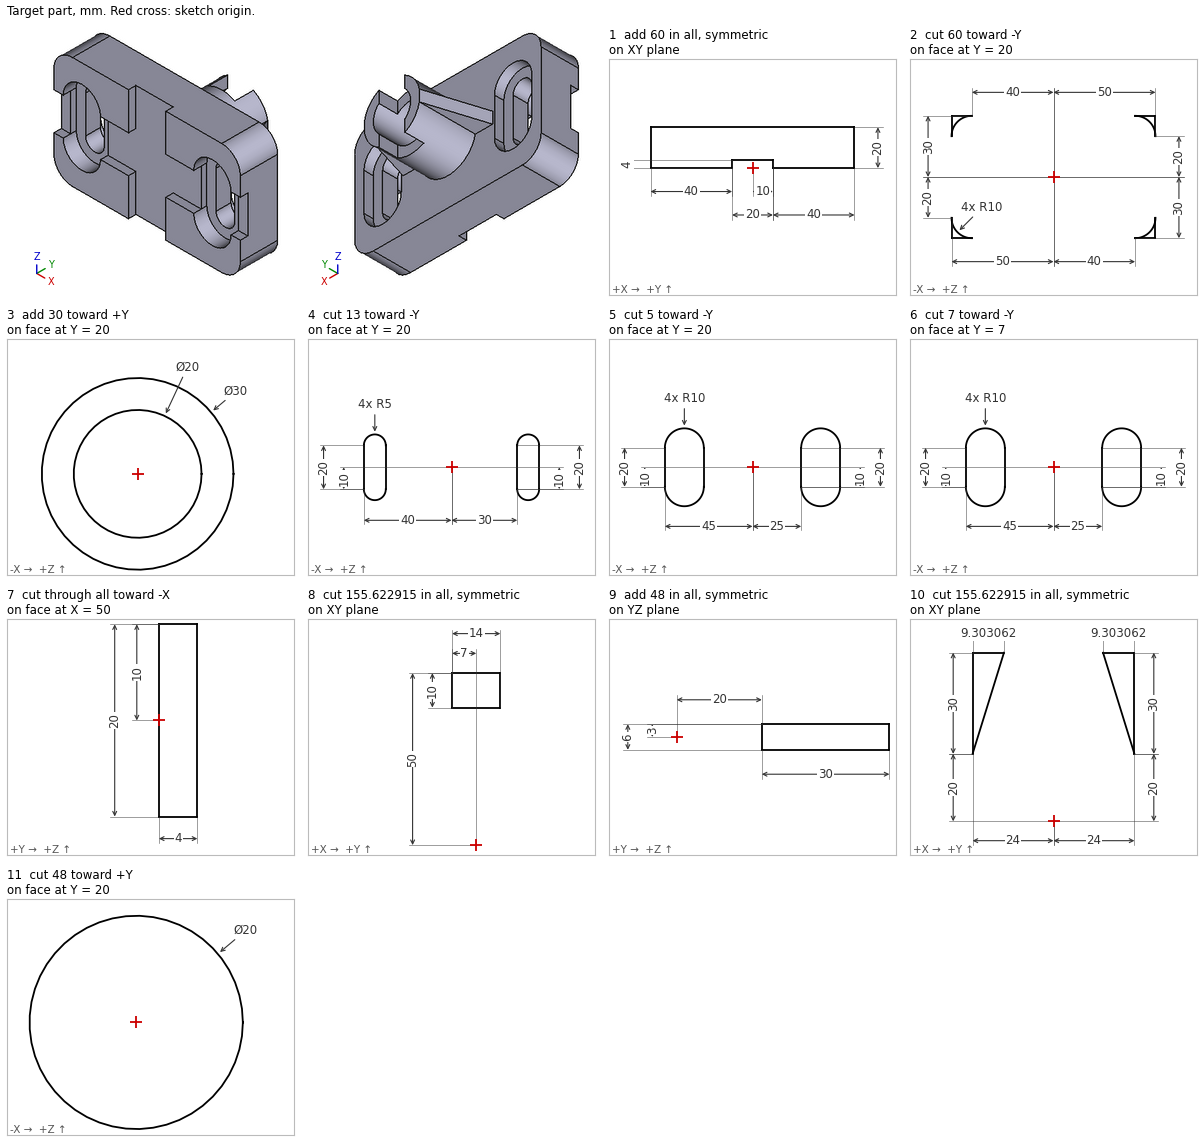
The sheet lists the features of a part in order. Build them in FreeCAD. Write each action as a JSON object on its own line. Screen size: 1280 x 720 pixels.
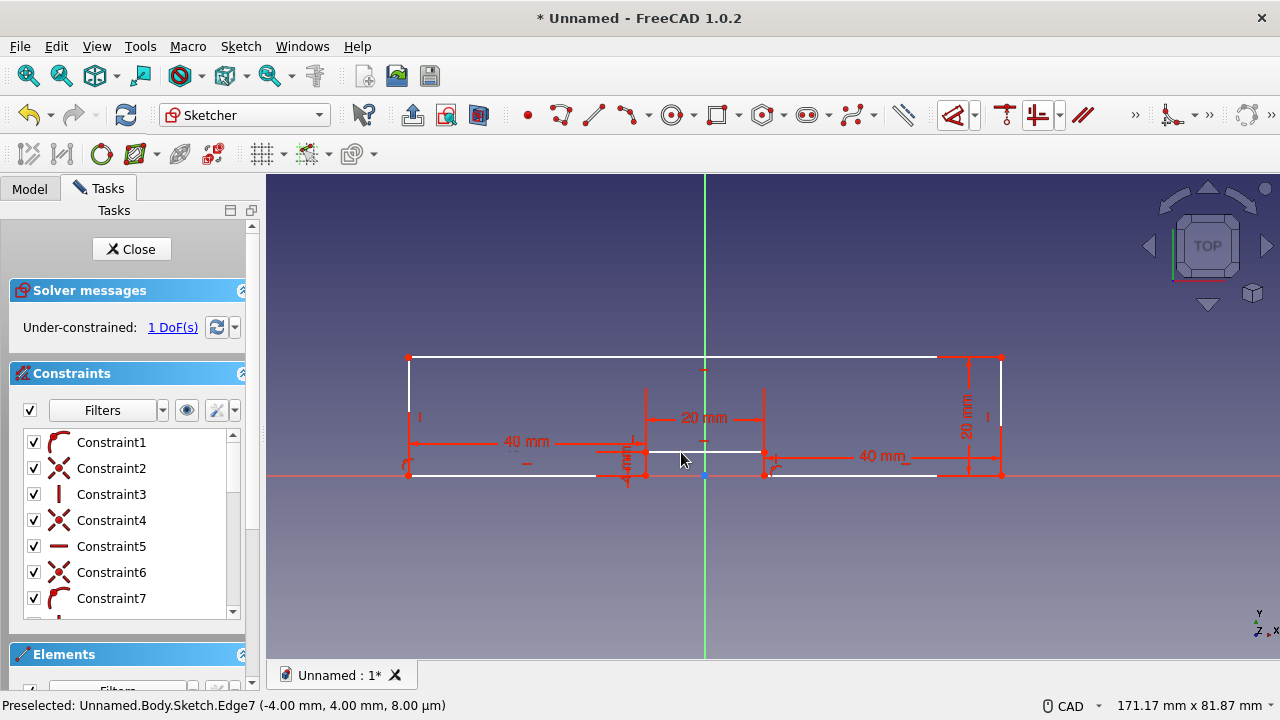
{"action": "left_click", "coordinate": [764, 476]}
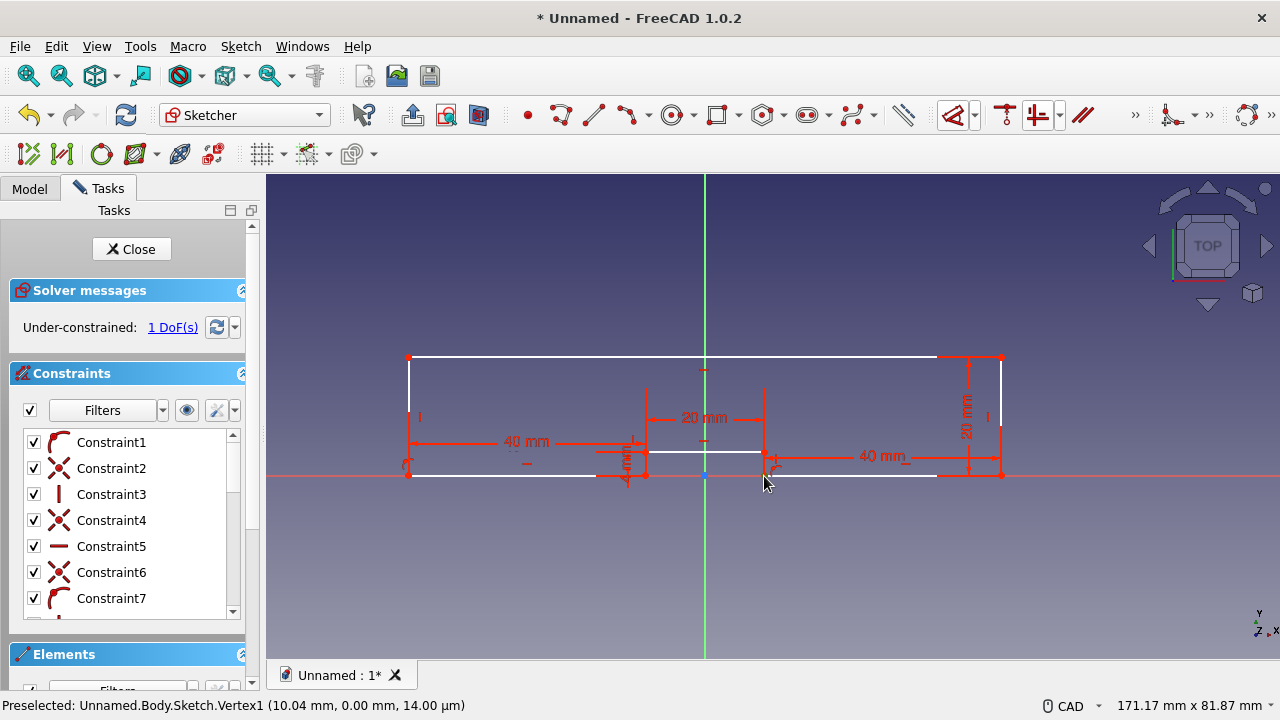
{"action": "key", "text": "l"}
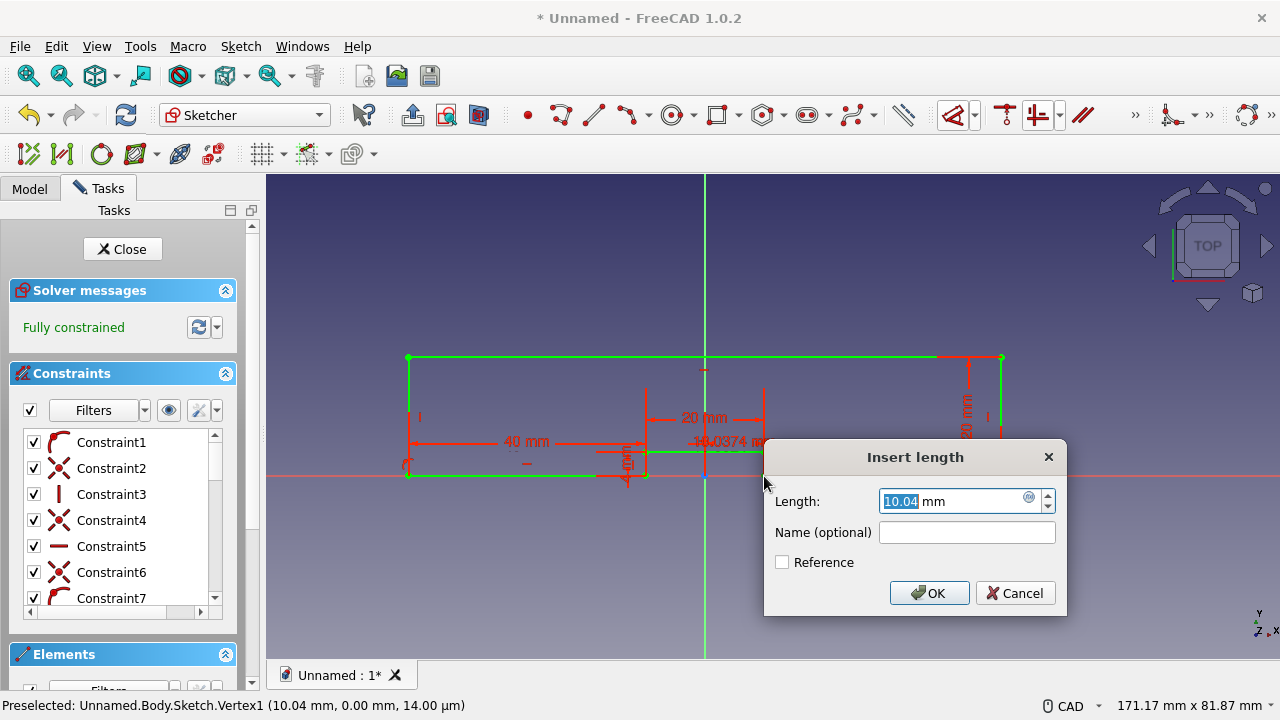
{"action": "type", "text": "10"}
{"action": "key", "text": "Return"}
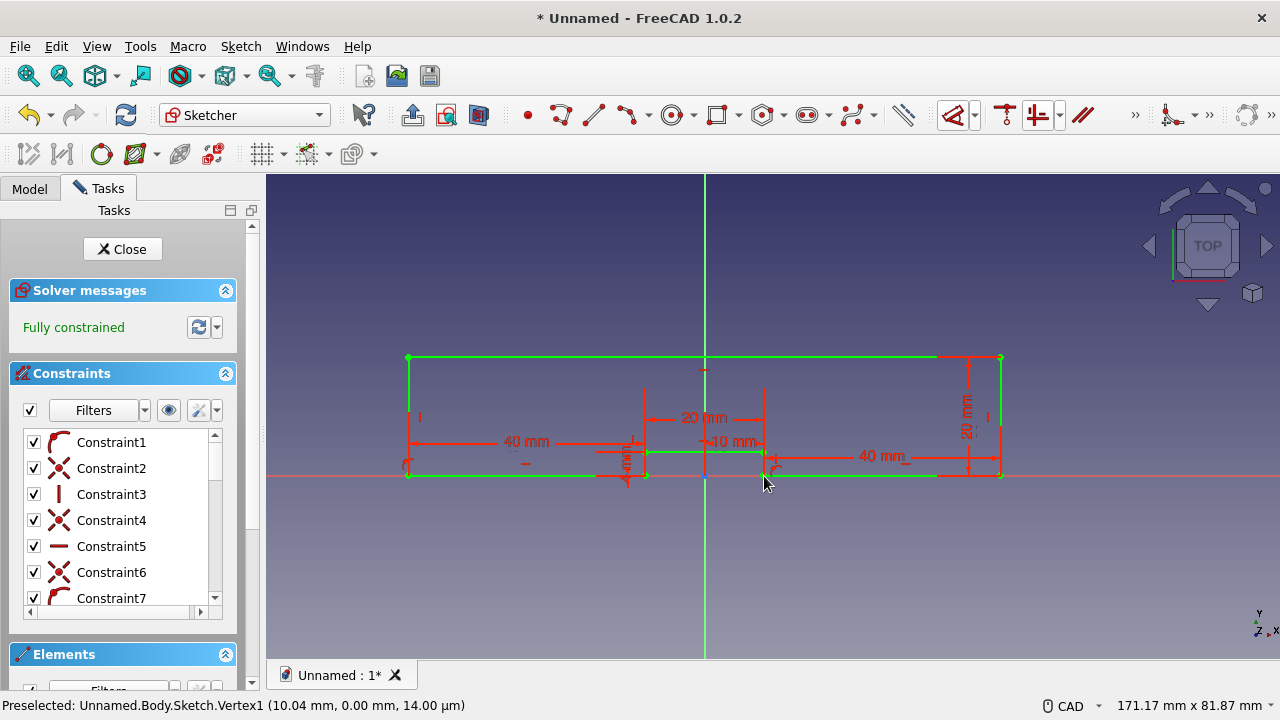
{"action": "left_click", "coordinate": [123, 249]}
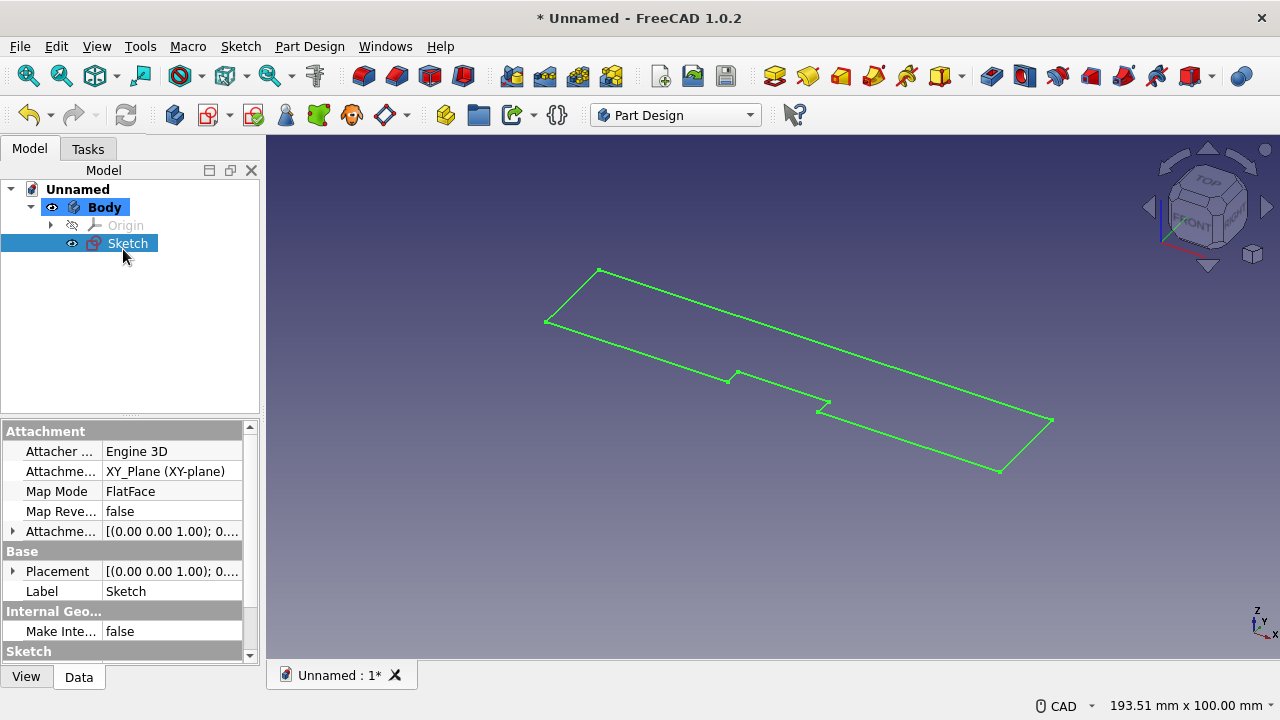
{"action": "left_click", "coordinate": [775, 76]}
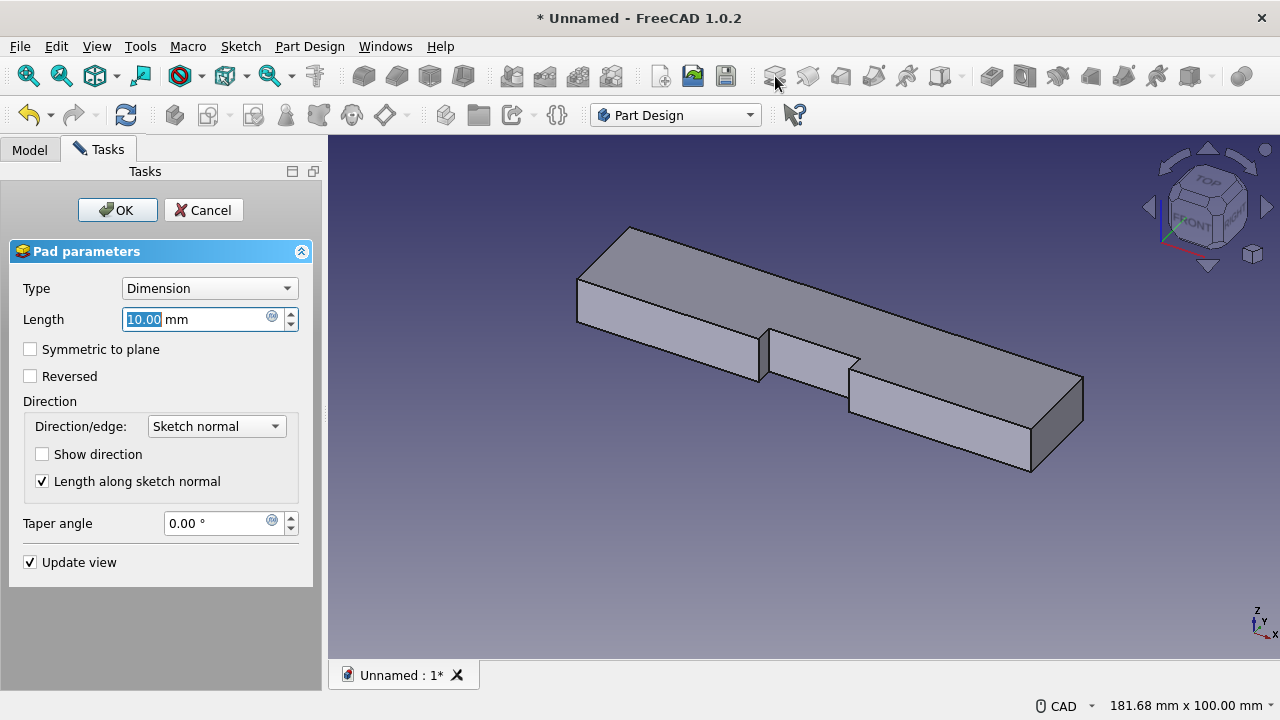
{"action": "type", "text": "60"}
{"action": "key", "text": "Tab"}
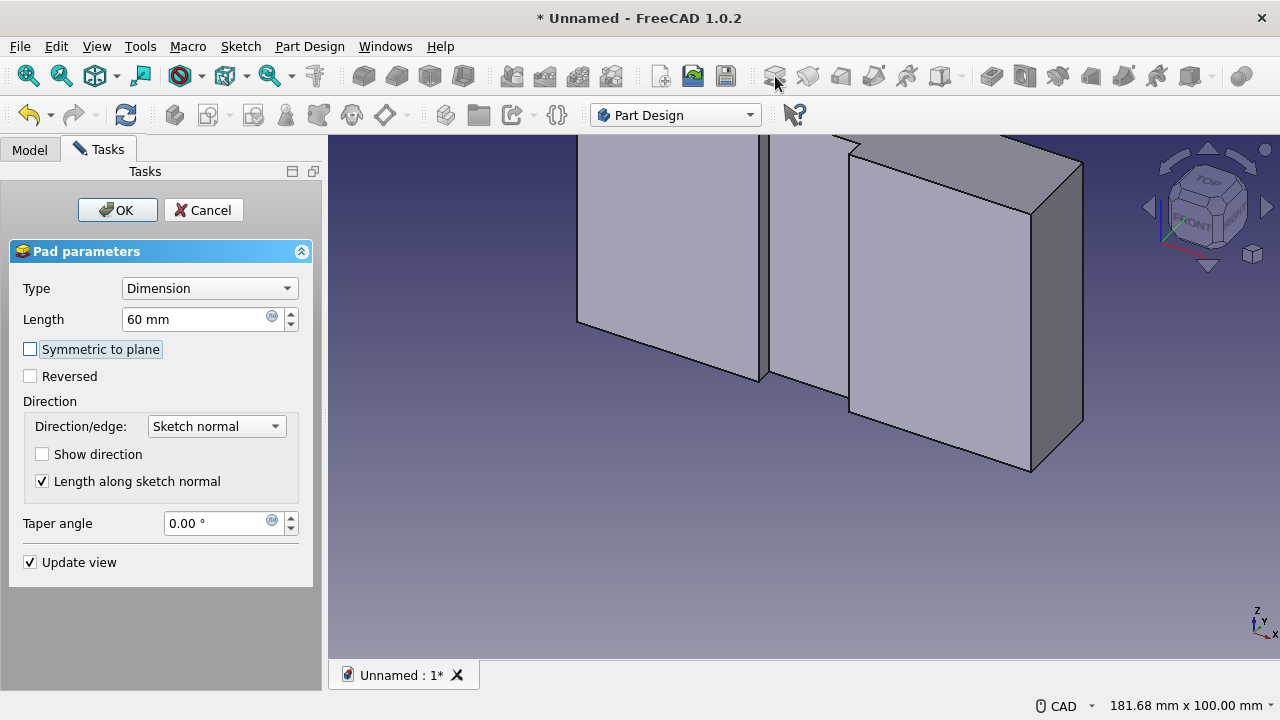
{"action": "left_click", "coordinate": [31, 349]}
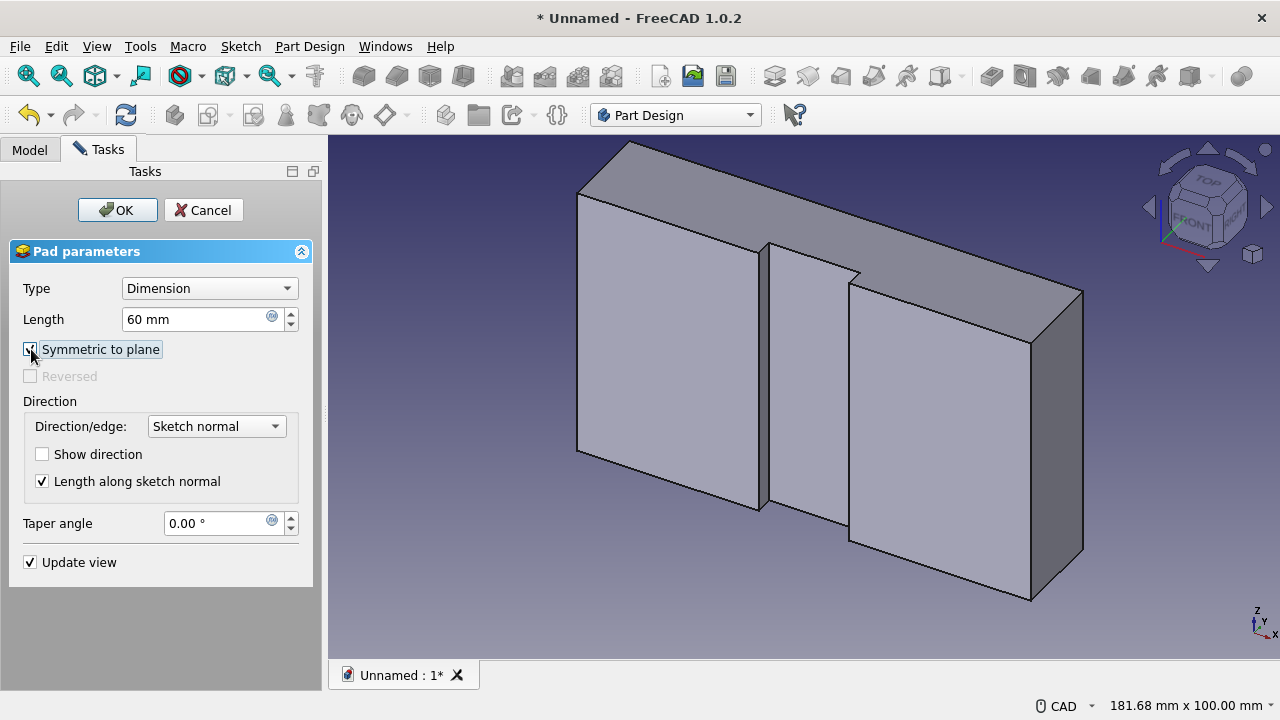
{"action": "left_click", "coordinate": [118, 210]}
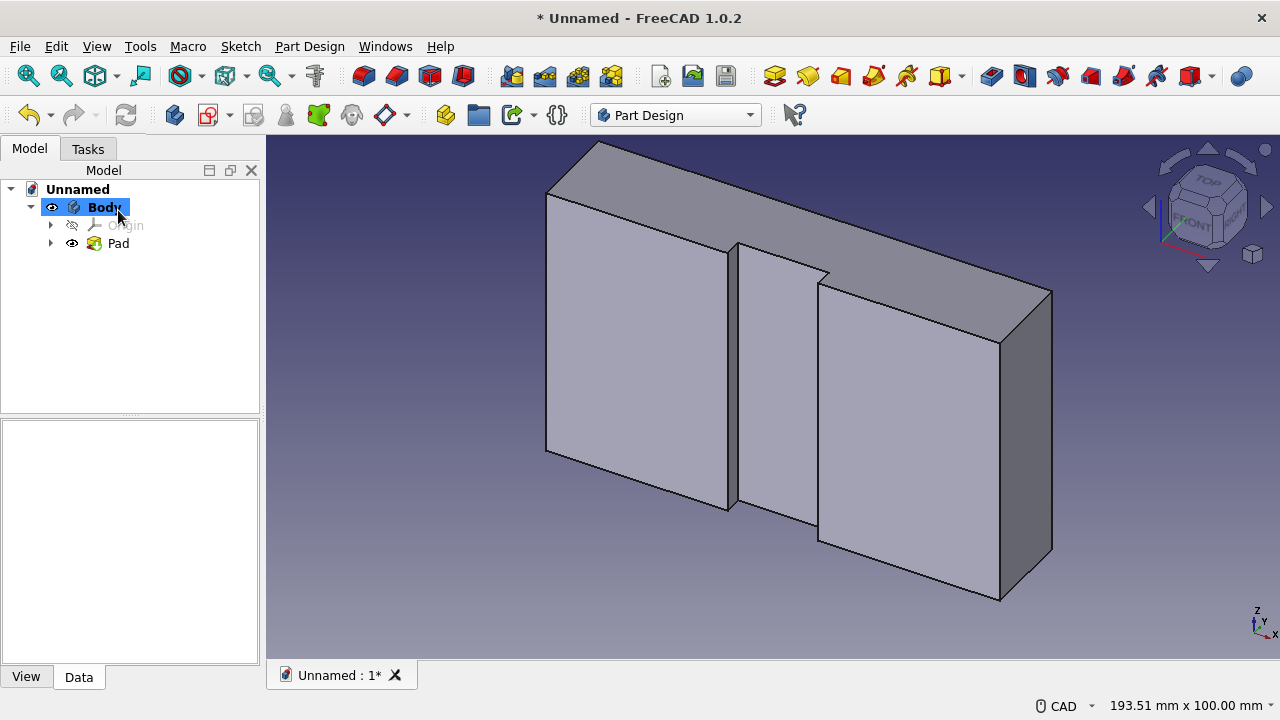
{"action": "key", "text": "4"}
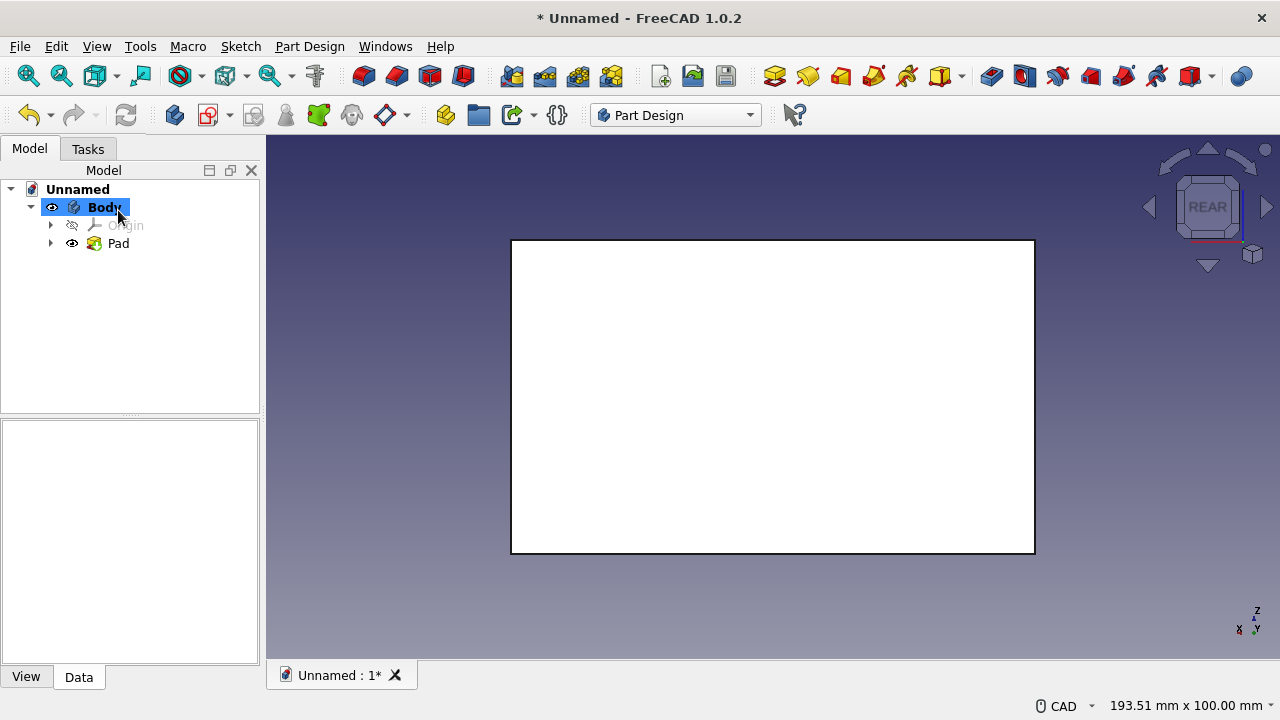
{"action": "left_click", "coordinate": [698, 396]}